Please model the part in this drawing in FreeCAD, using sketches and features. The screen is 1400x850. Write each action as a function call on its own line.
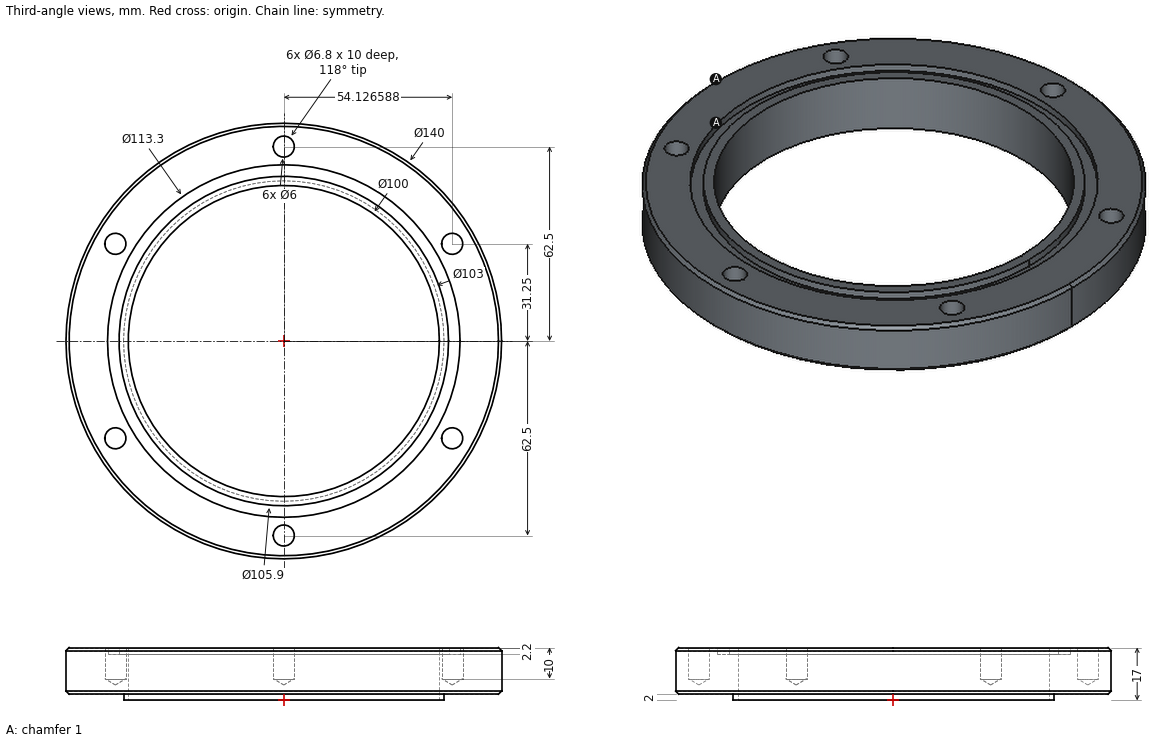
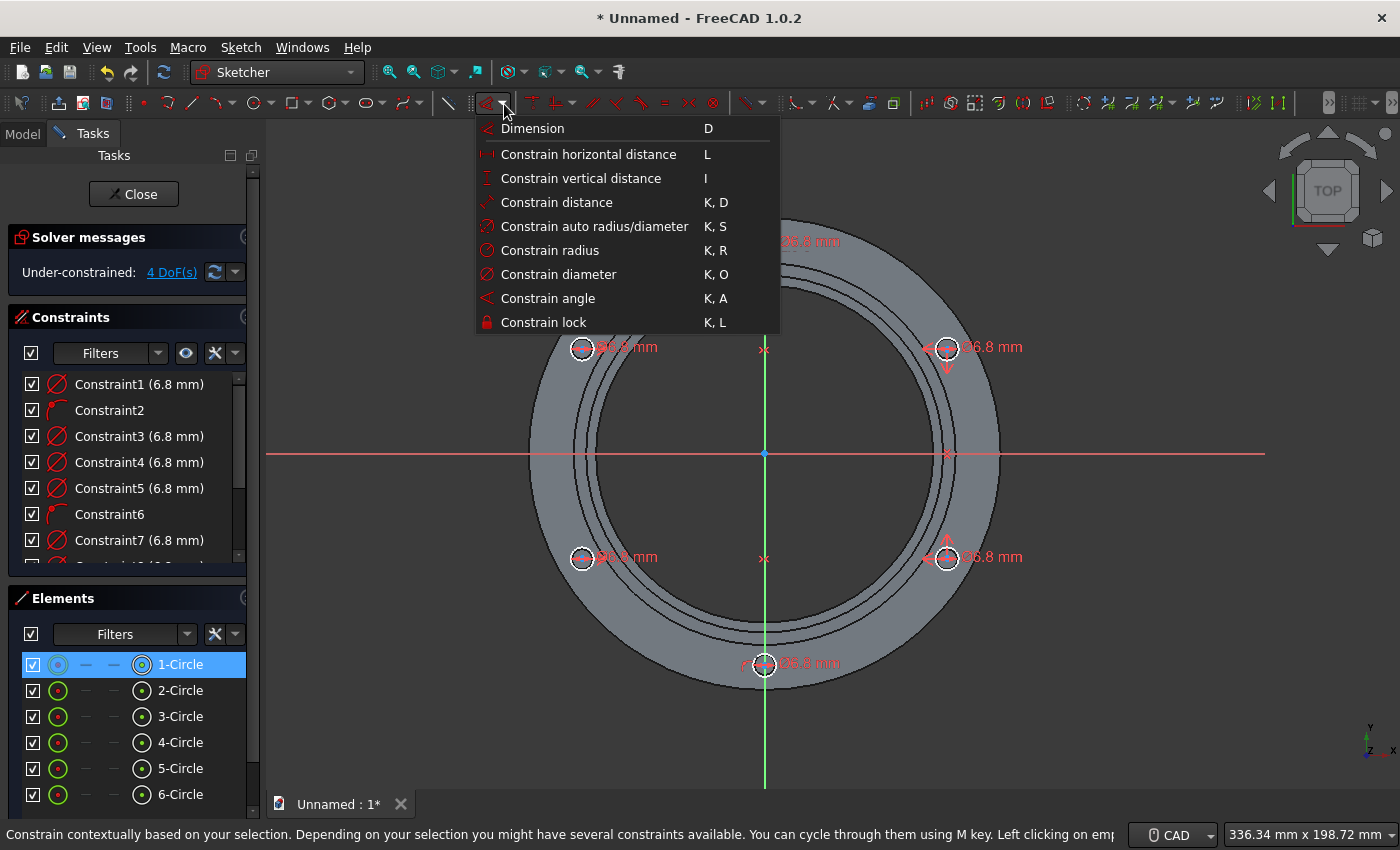
click(628, 178)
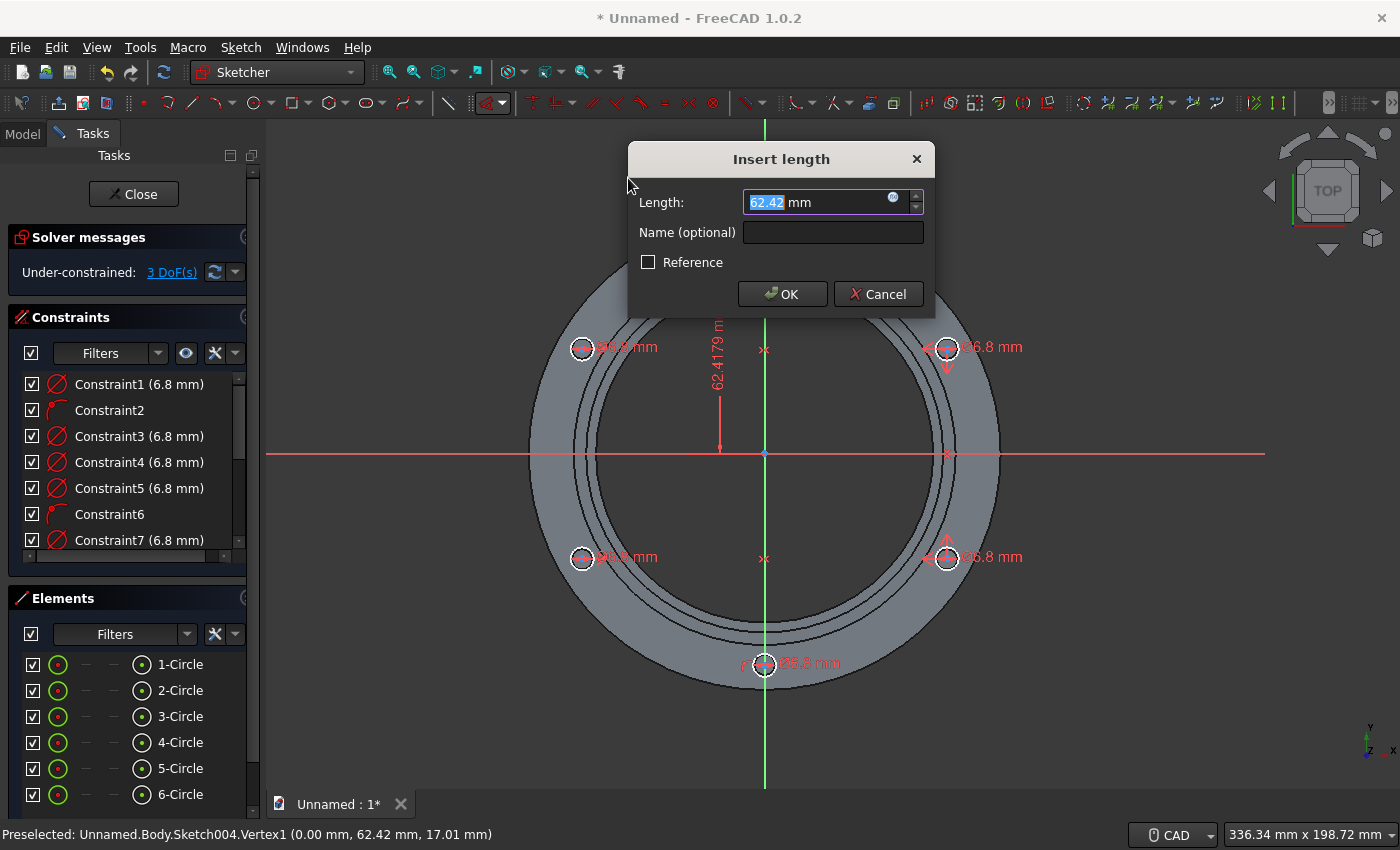
text(62.5)
key(Return)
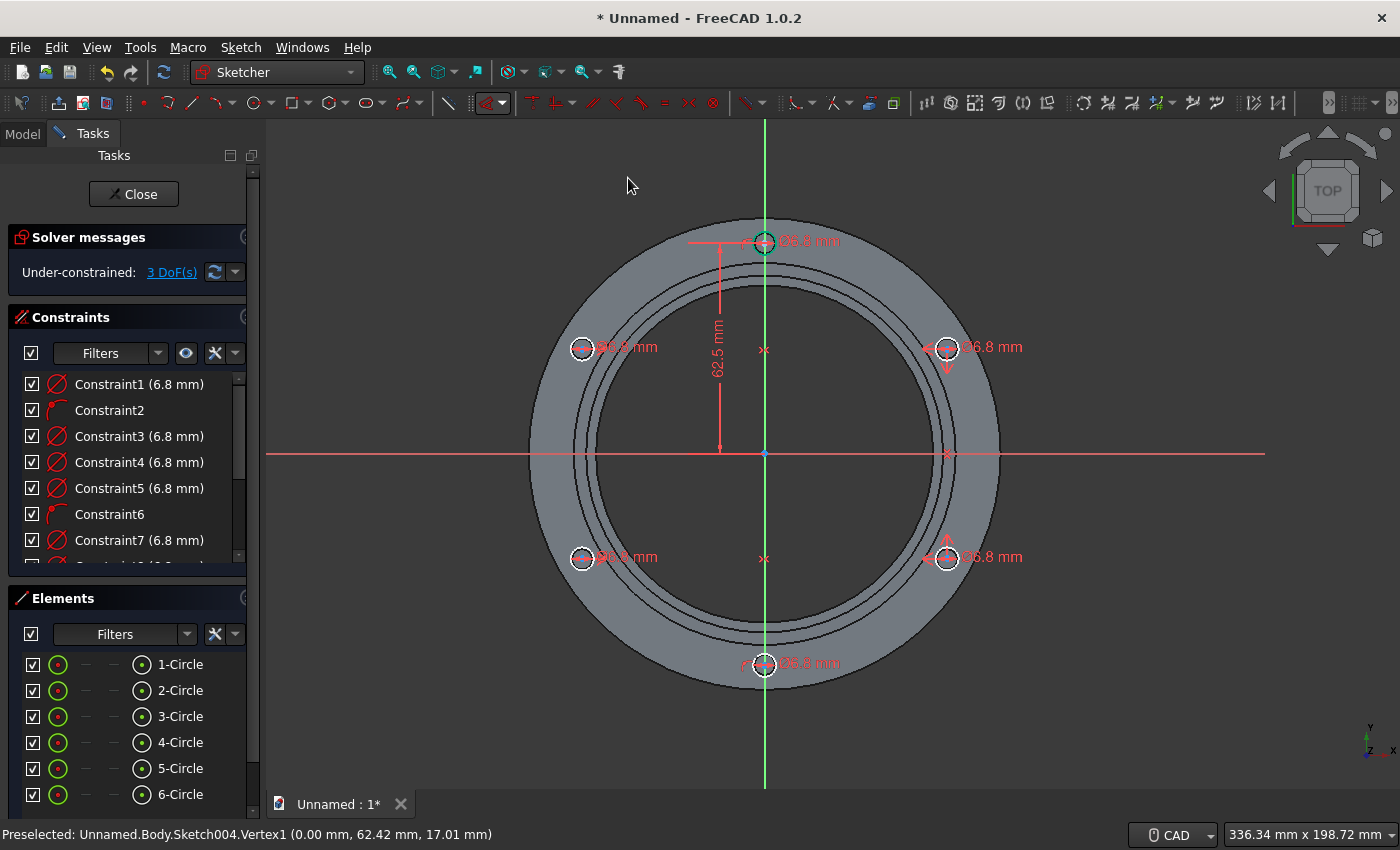
click(765, 665)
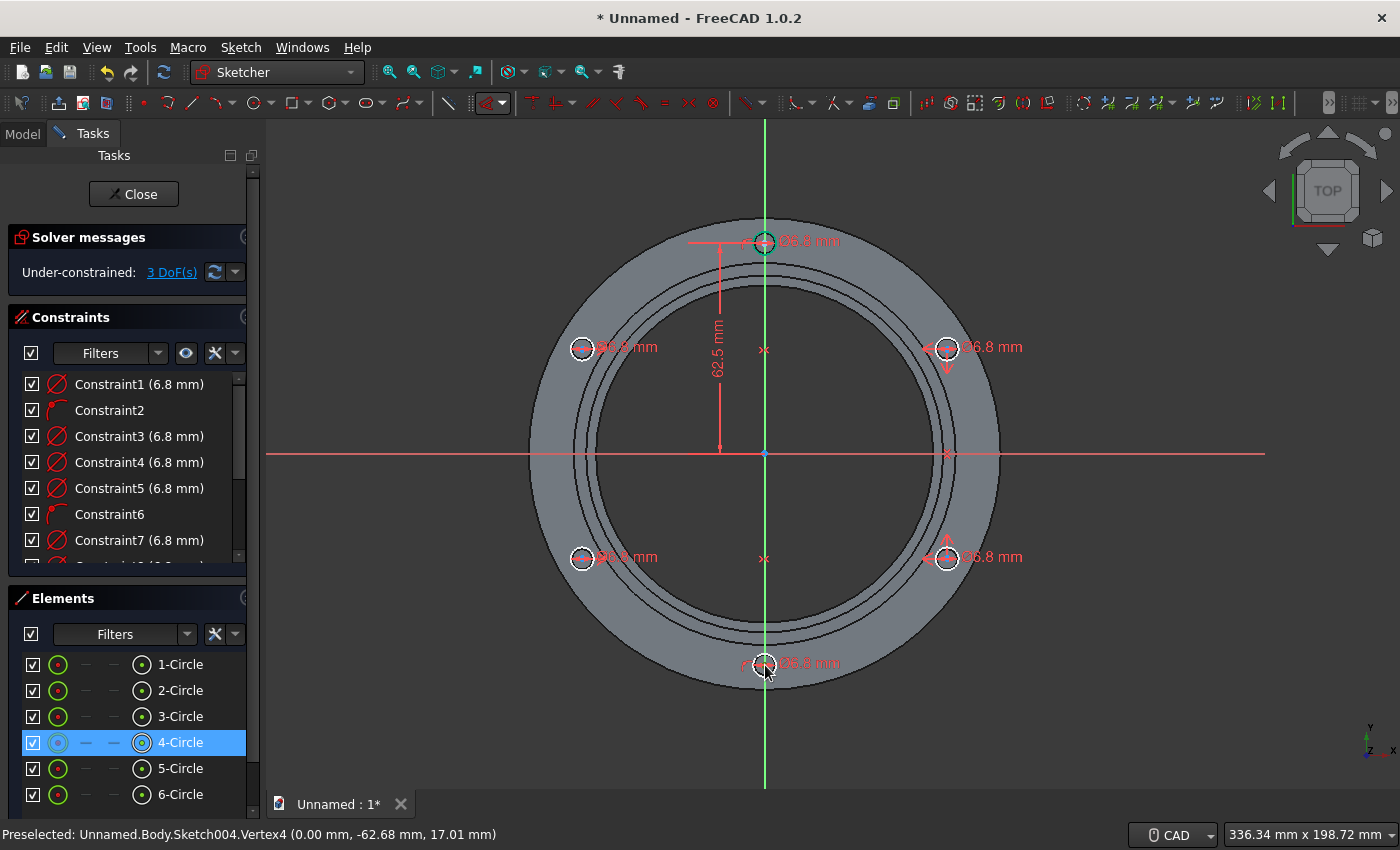
key(i)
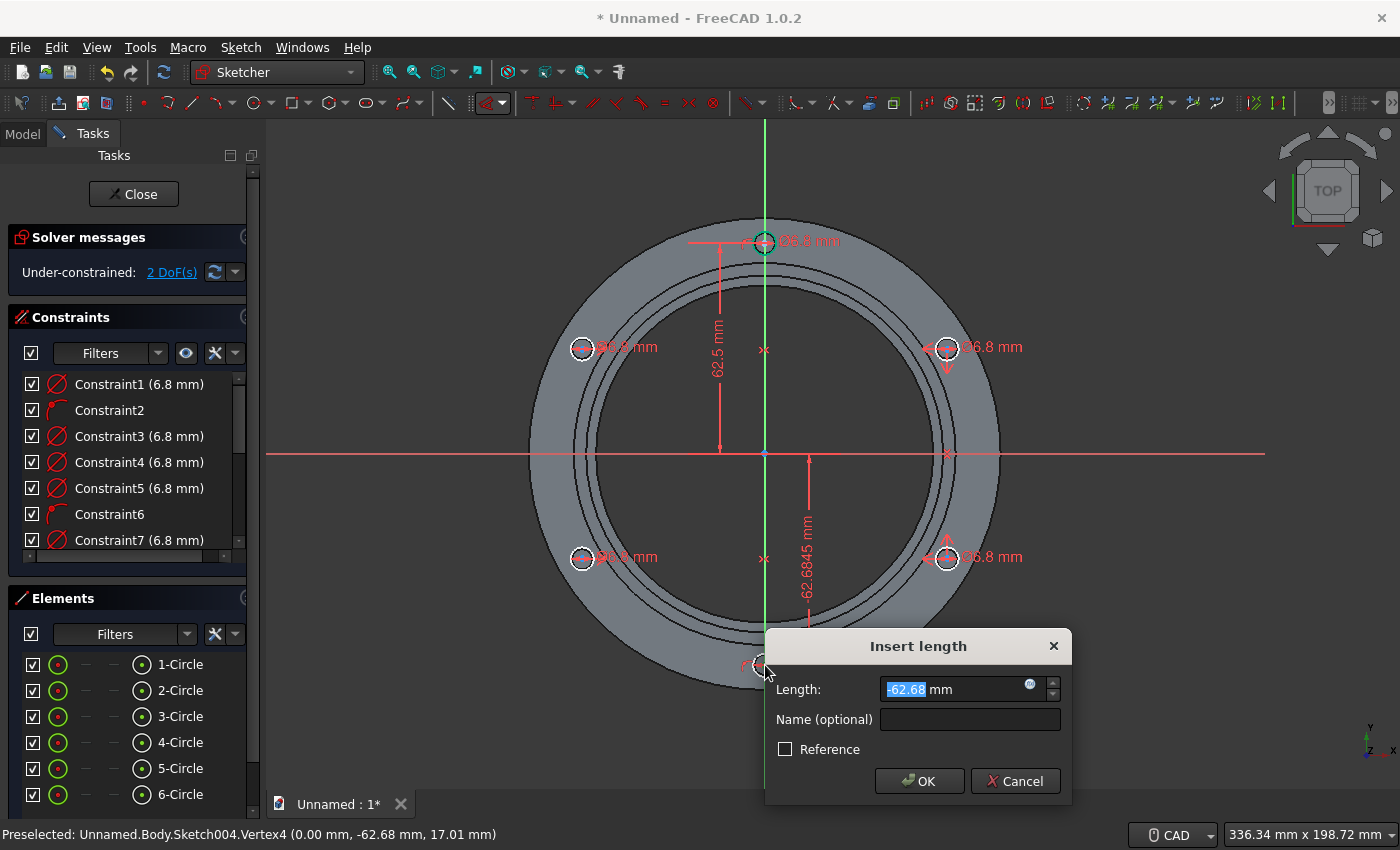
text(-62.5)
key(Return)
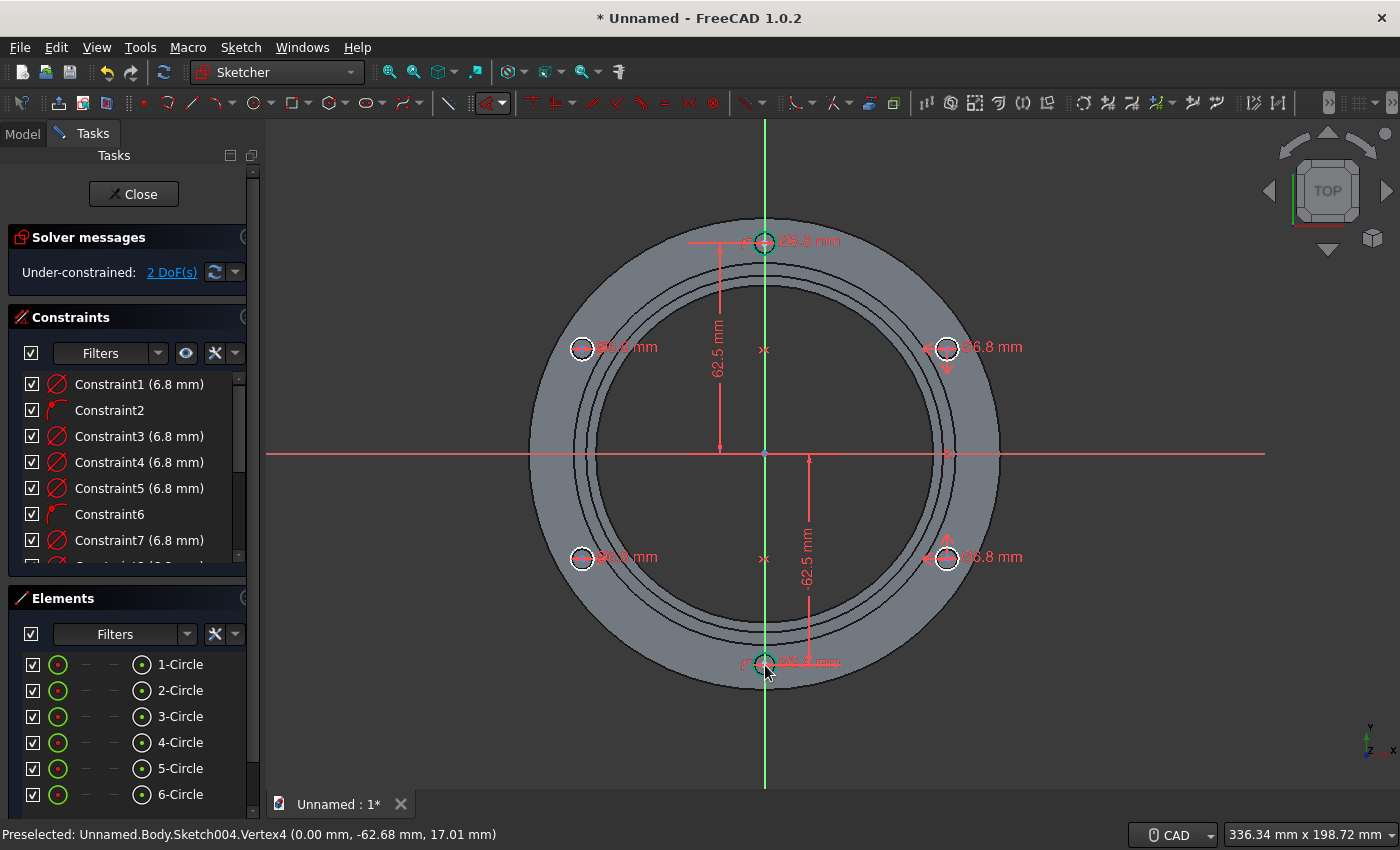
click(947, 349)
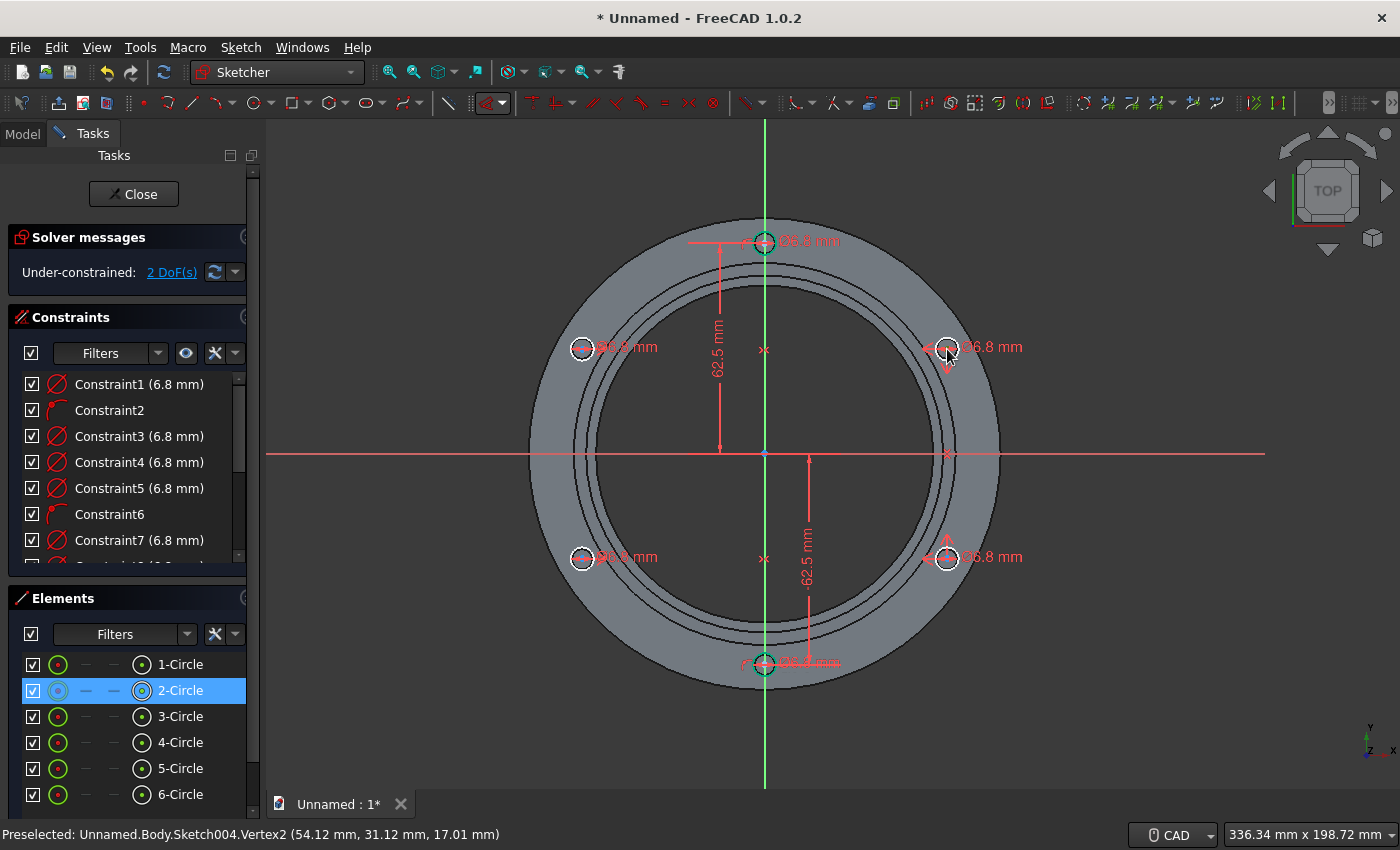
key(i)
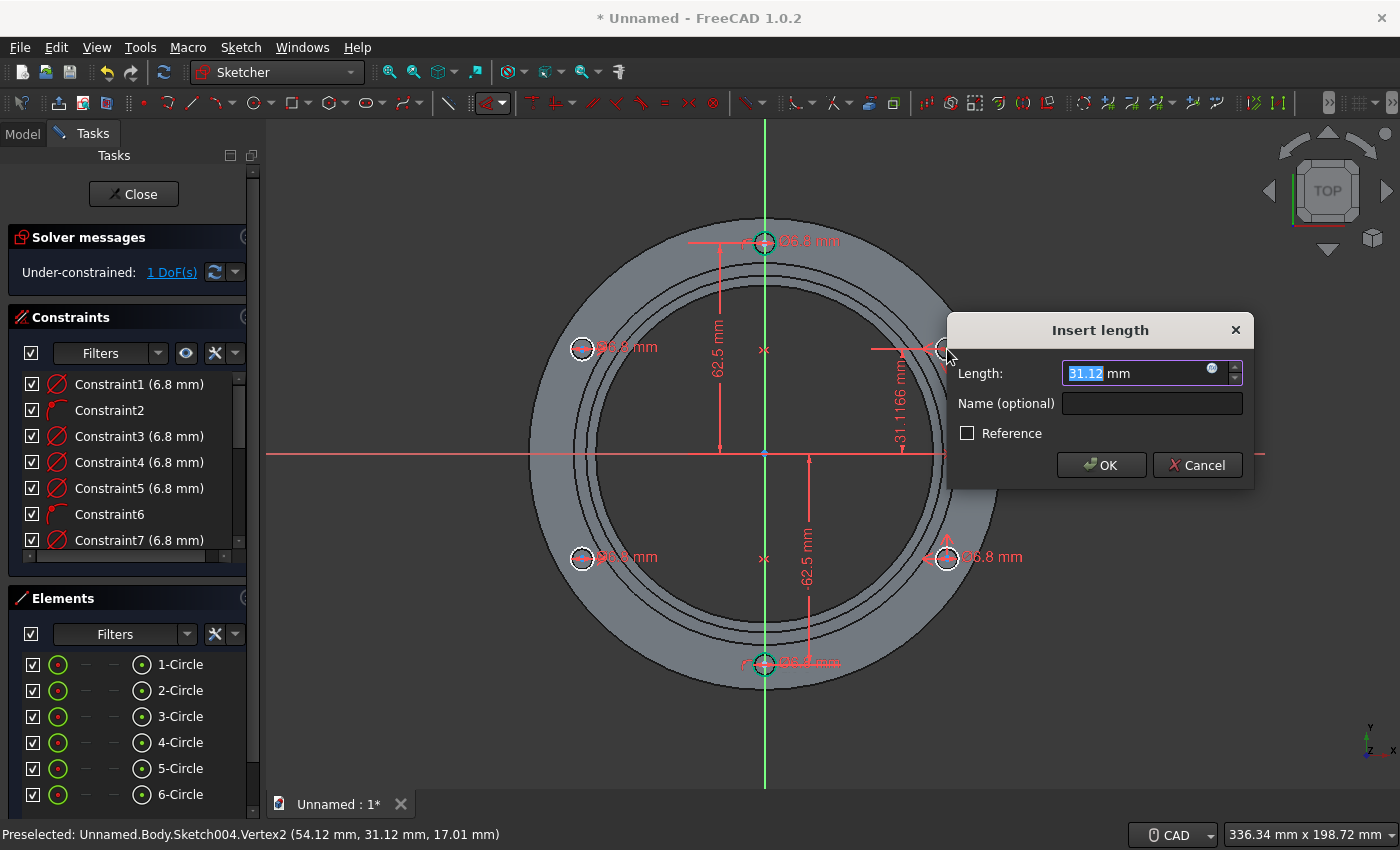
text(31.25)
key(Return)